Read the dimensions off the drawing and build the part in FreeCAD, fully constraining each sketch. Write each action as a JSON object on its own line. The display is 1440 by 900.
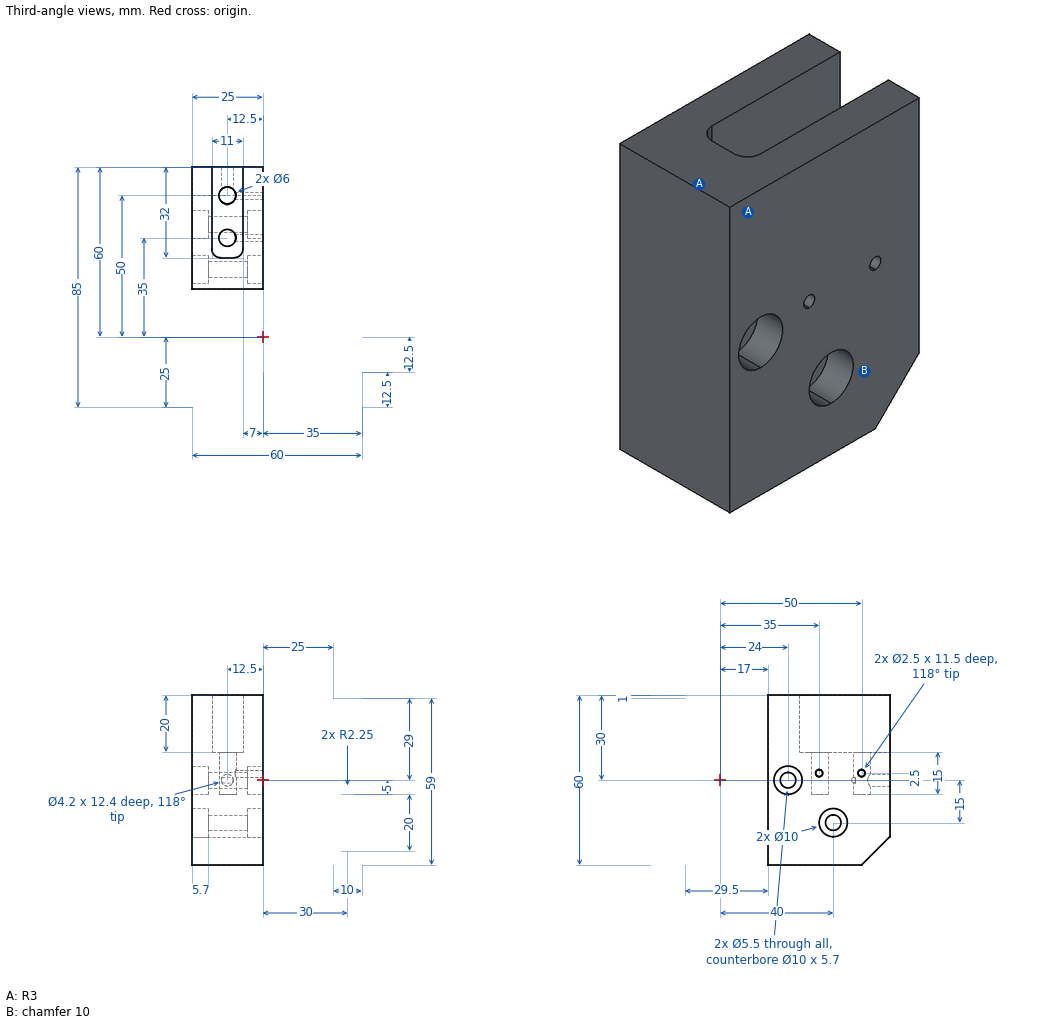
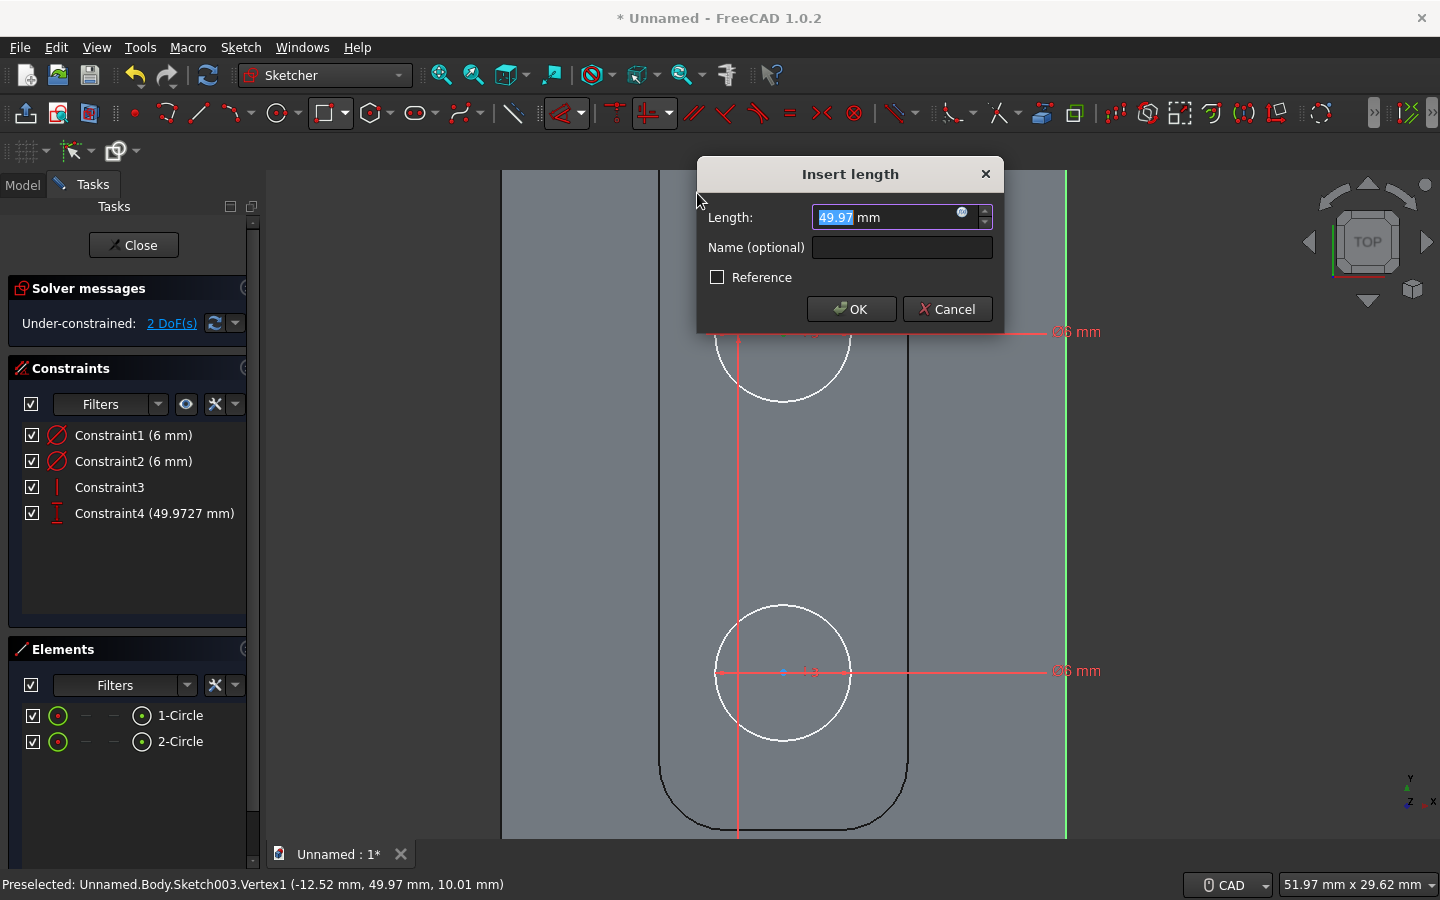
{"action": "type", "text": "50"}
{"action": "key", "text": "Return"}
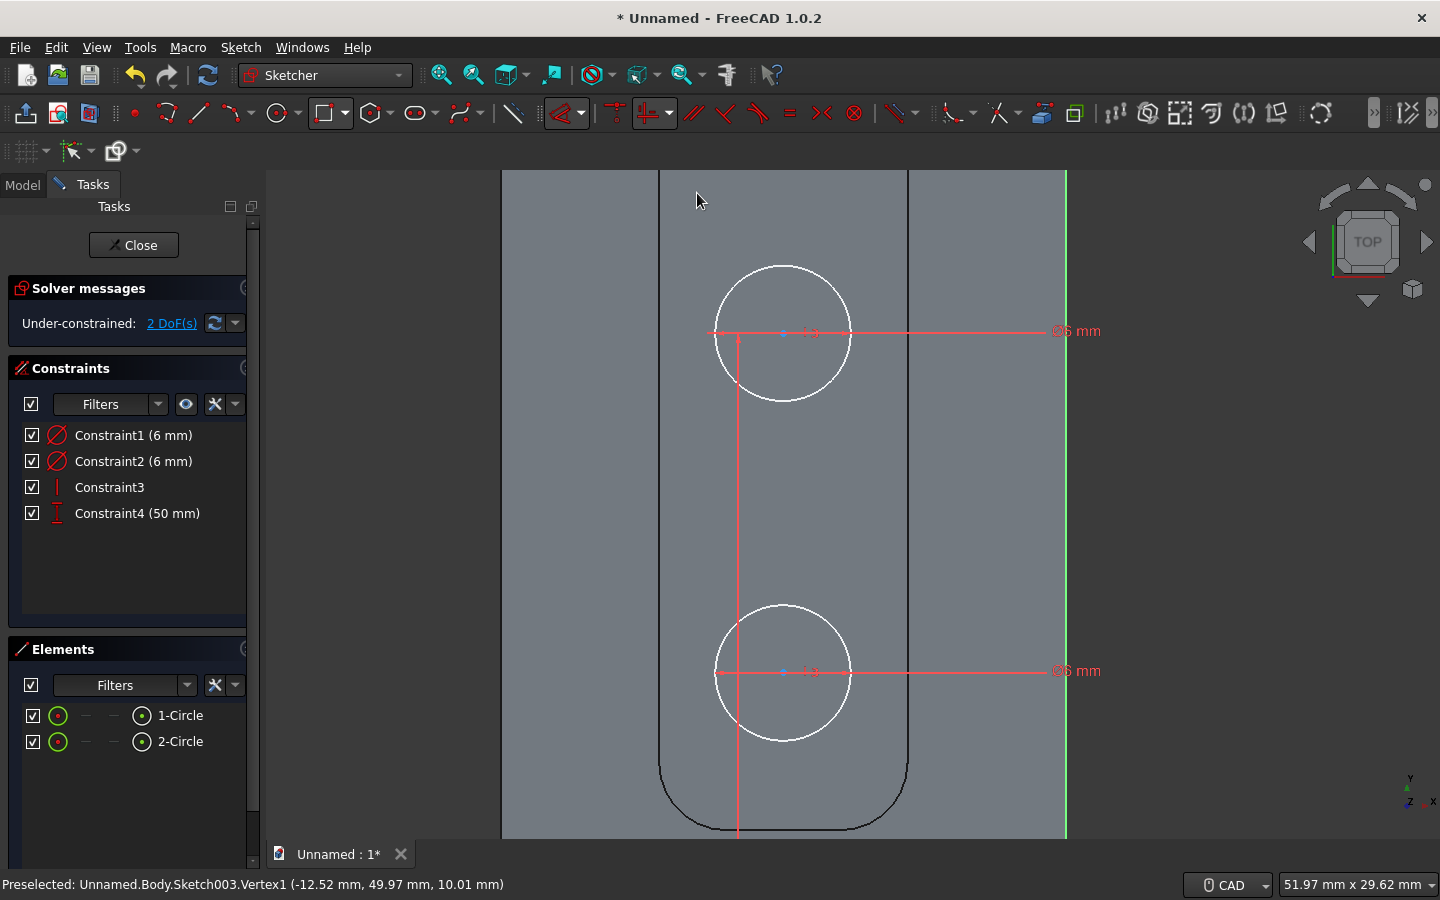
{"action": "left_click", "coordinate": [783, 673]}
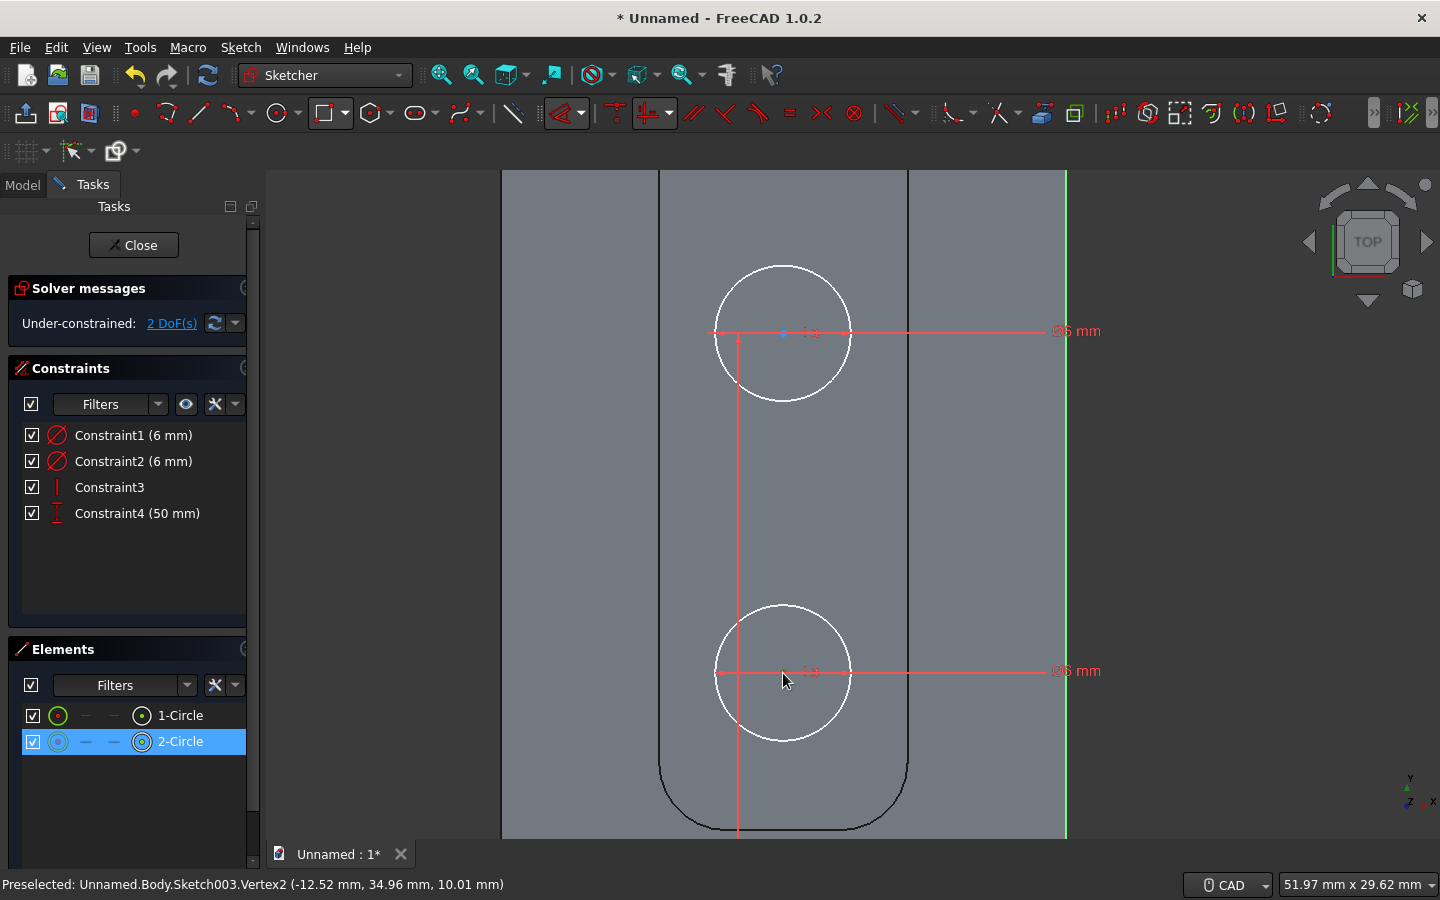
{"action": "key", "text": "i"}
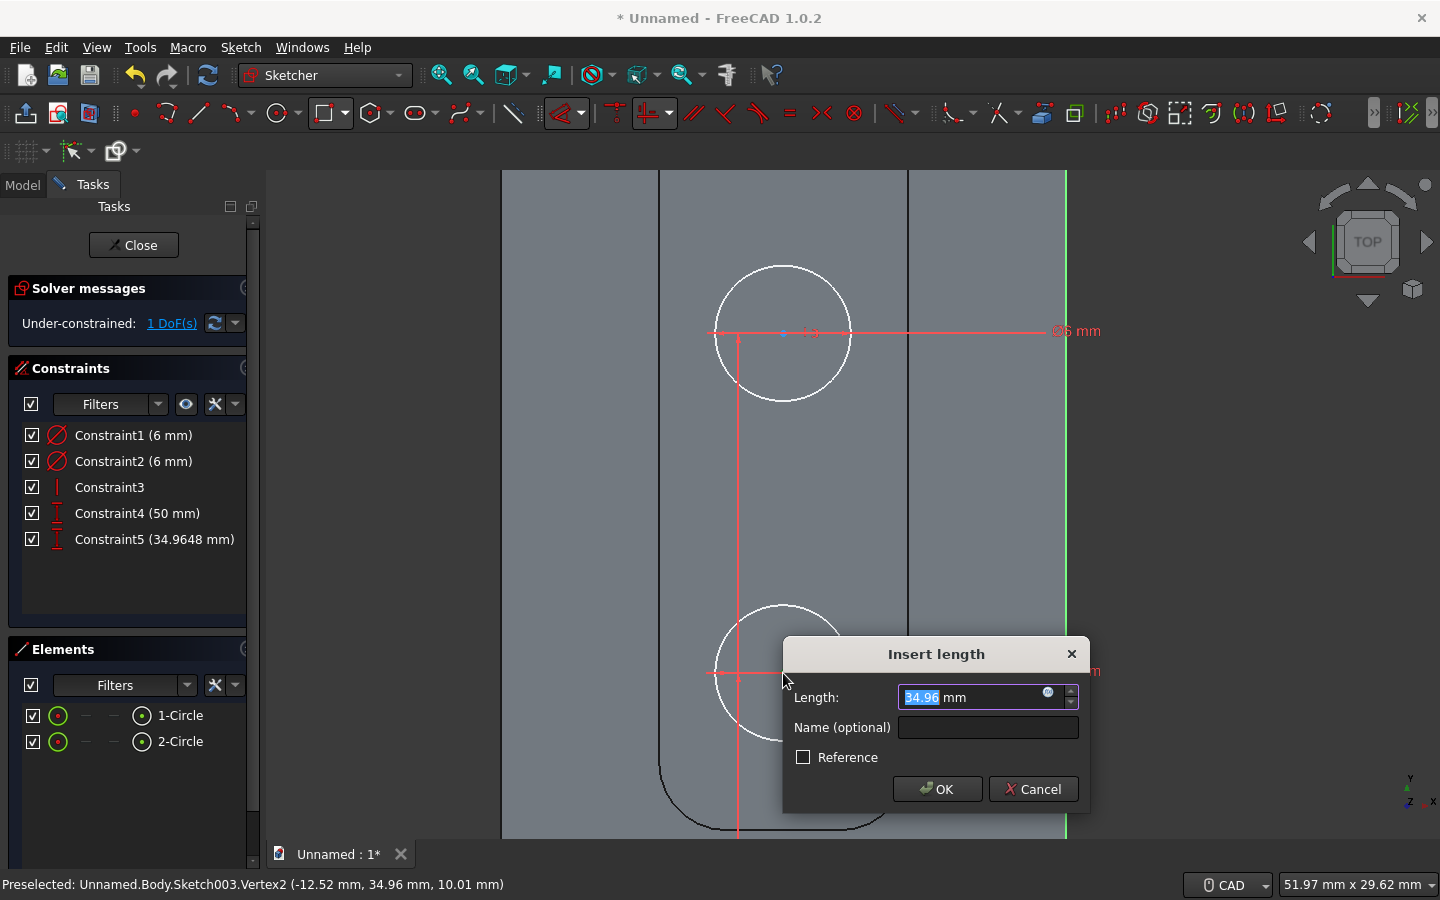
{"action": "type", "text": "35"}
{"action": "key", "text": "Return"}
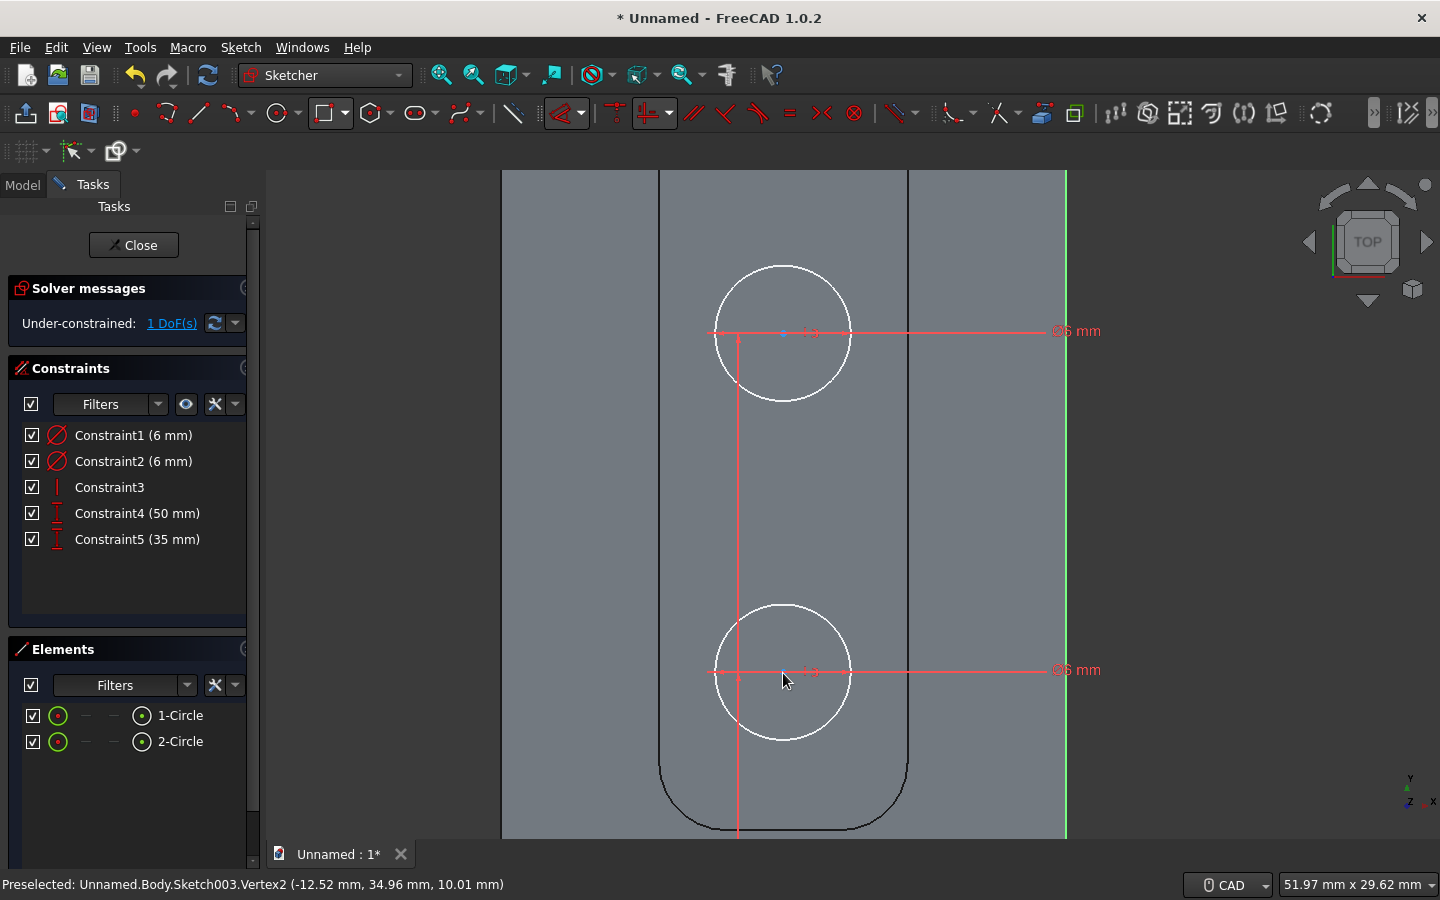
{"action": "left_click", "coordinate": [783, 333]}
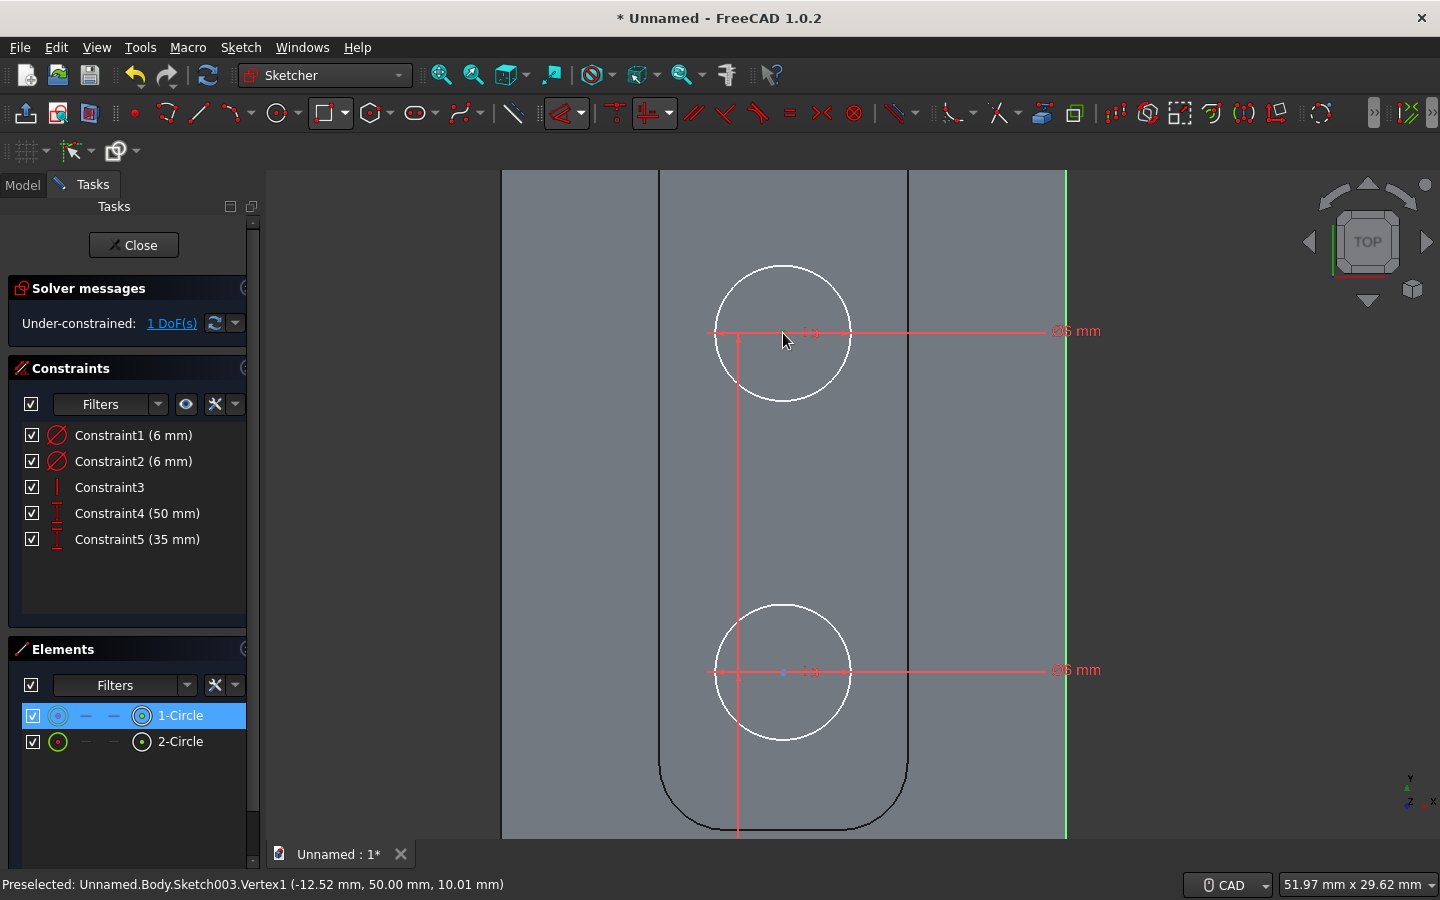
{"action": "left_click", "coordinate": [584, 114]}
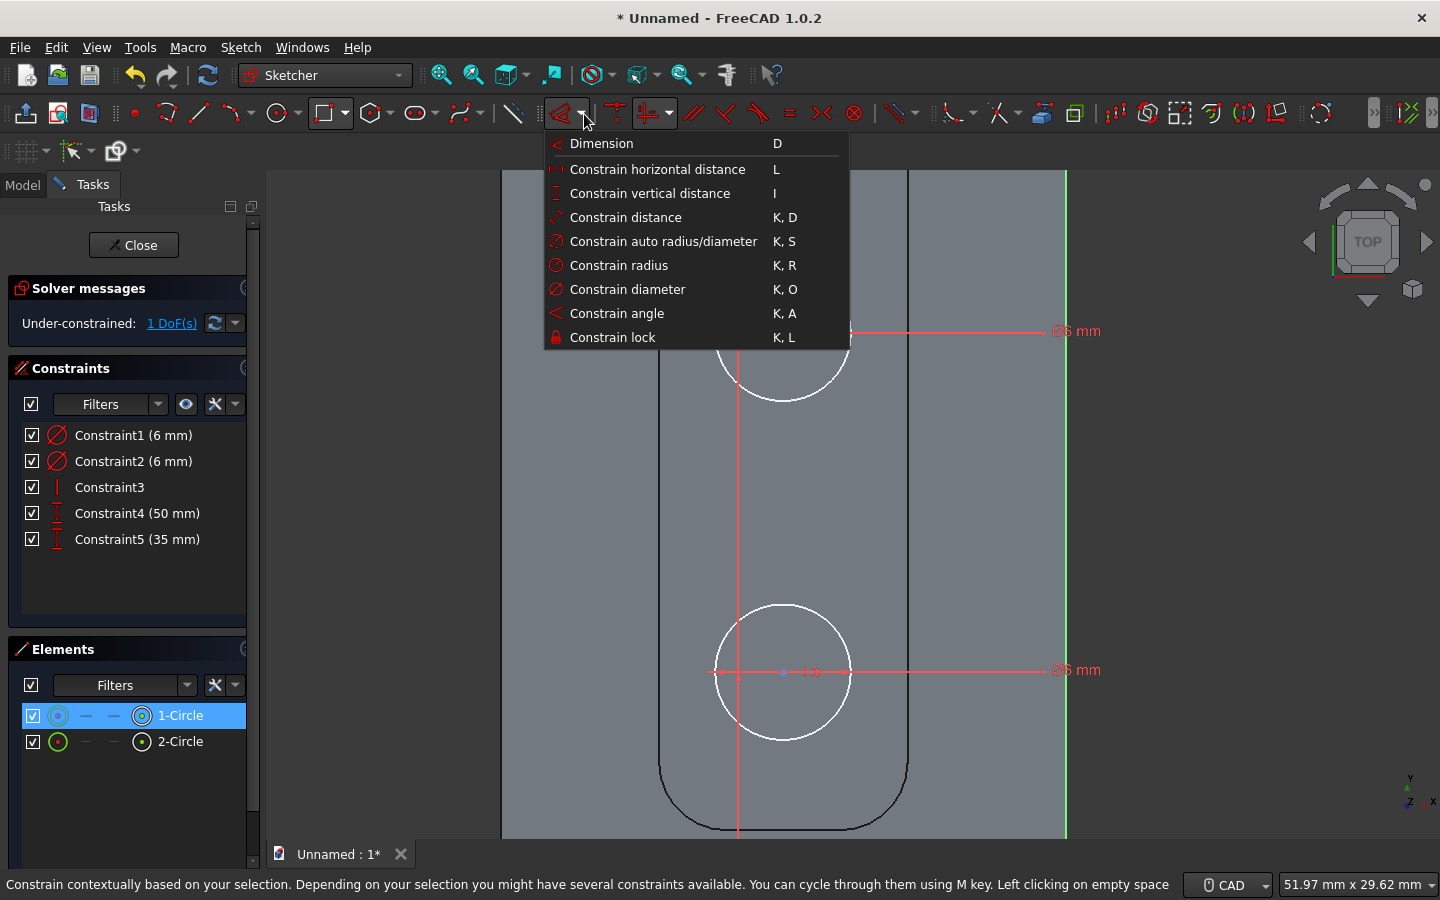
{"action": "left_click", "coordinate": [697, 169]}